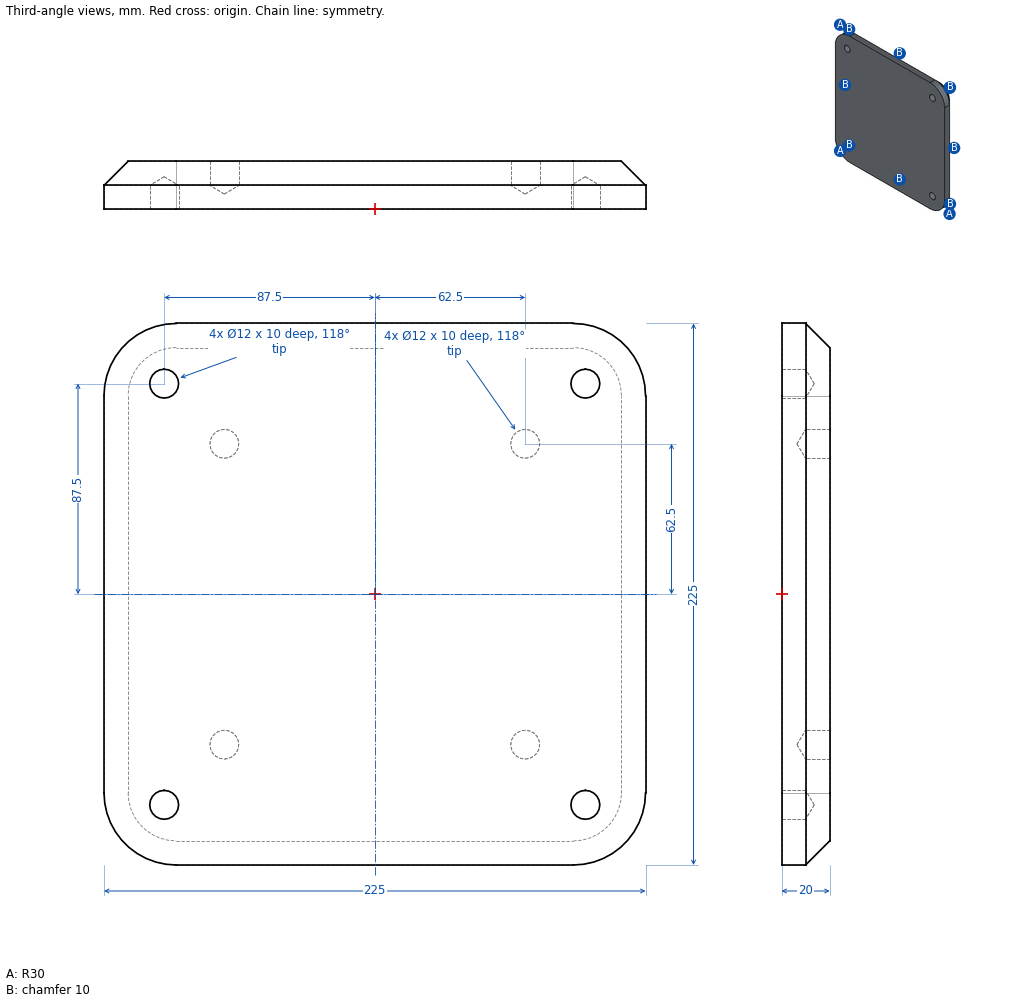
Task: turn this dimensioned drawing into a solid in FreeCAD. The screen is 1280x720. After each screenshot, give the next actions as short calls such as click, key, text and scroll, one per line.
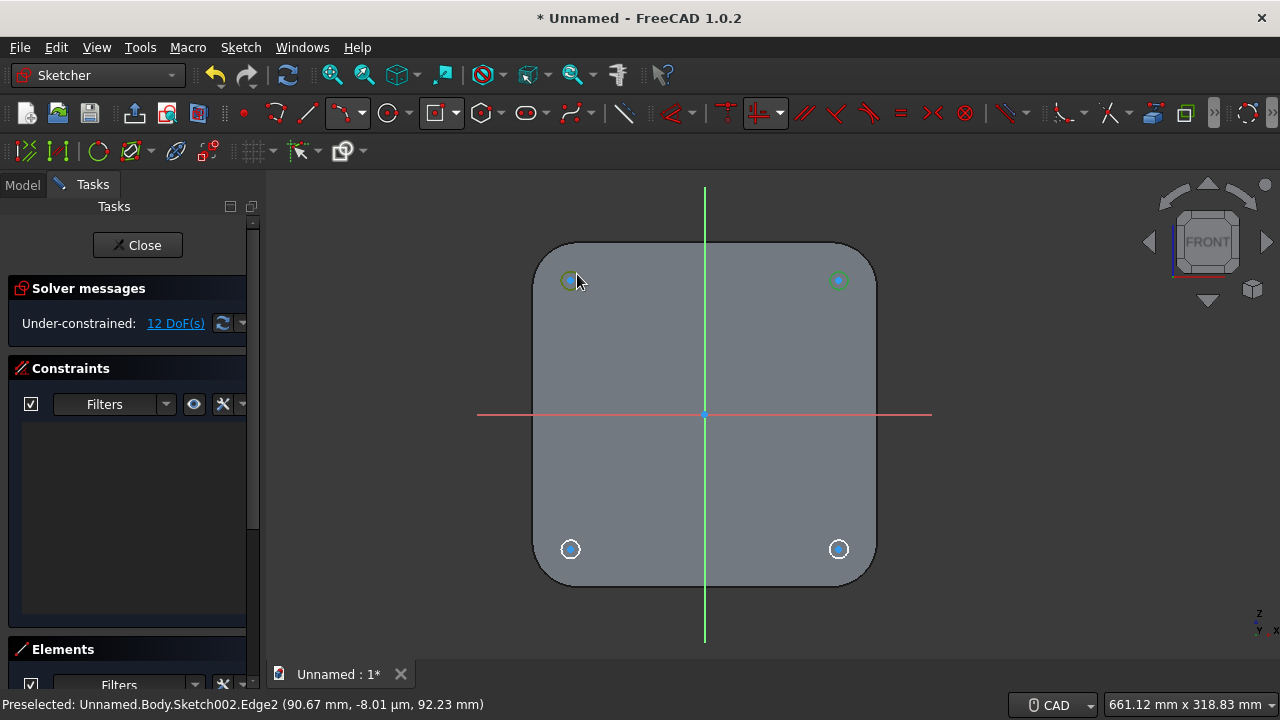
scroll(845, 543, up, 3)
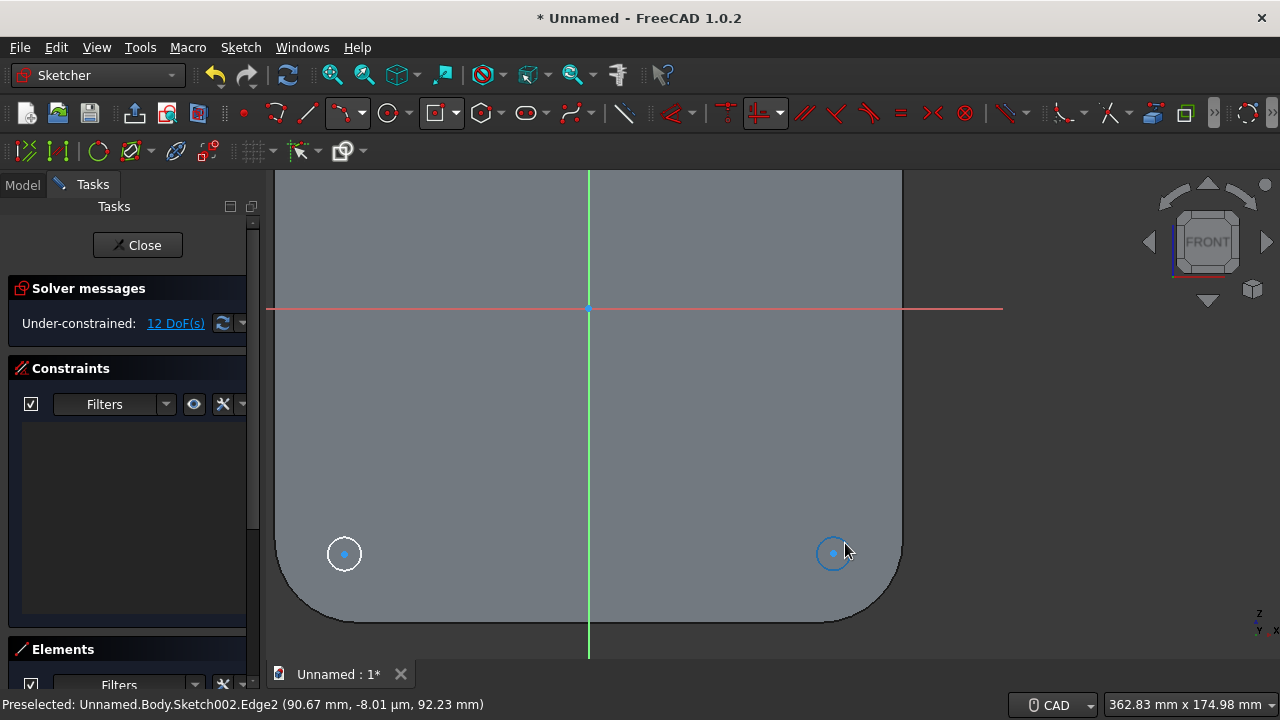
click(845, 542)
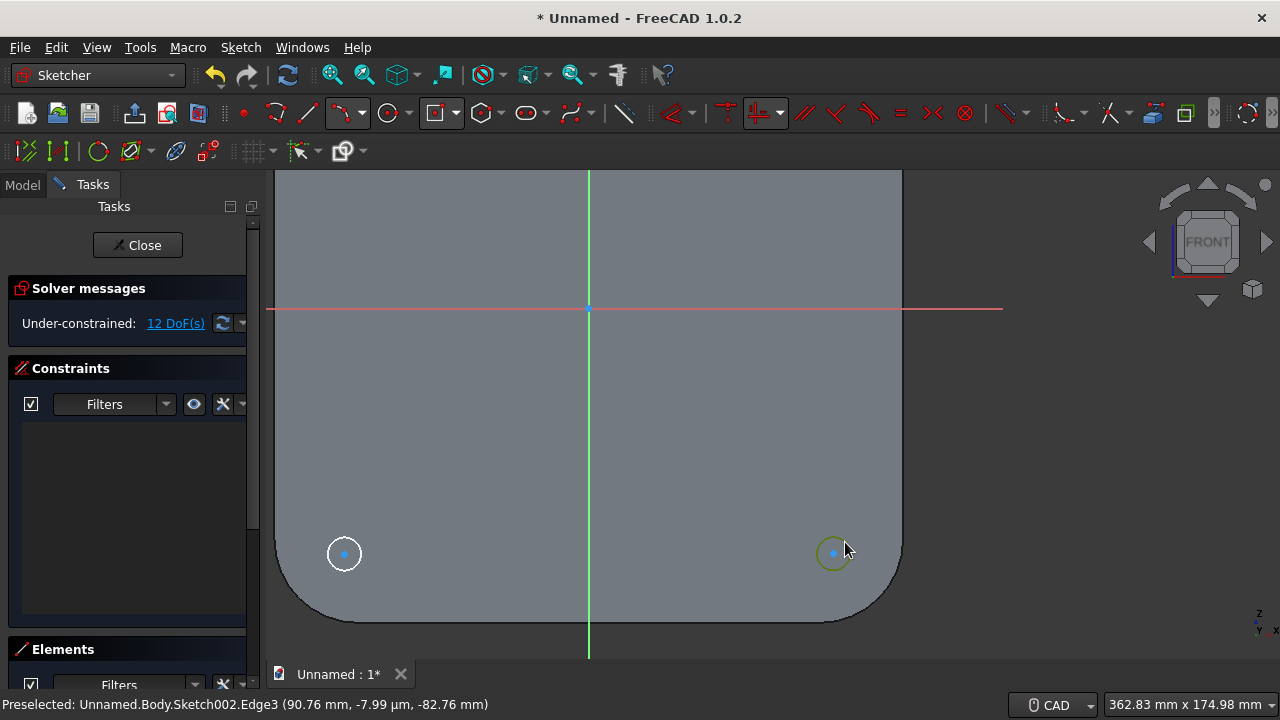
click(356, 542)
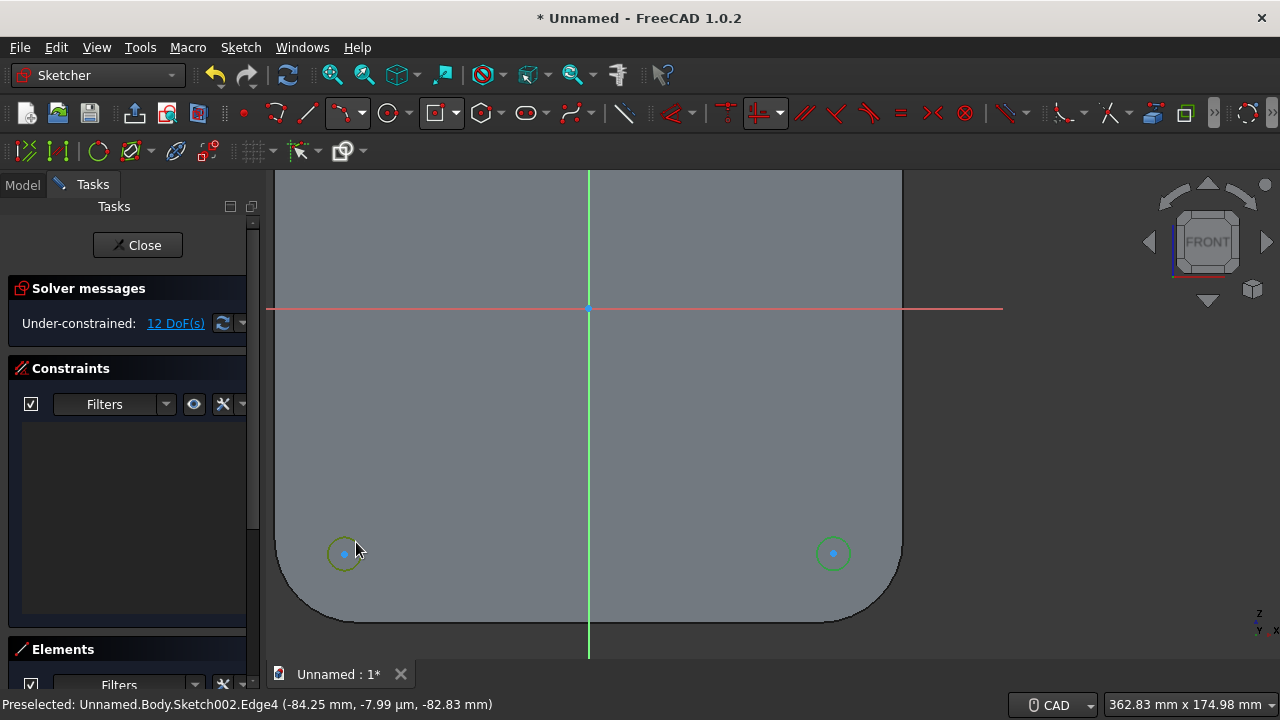
key(e)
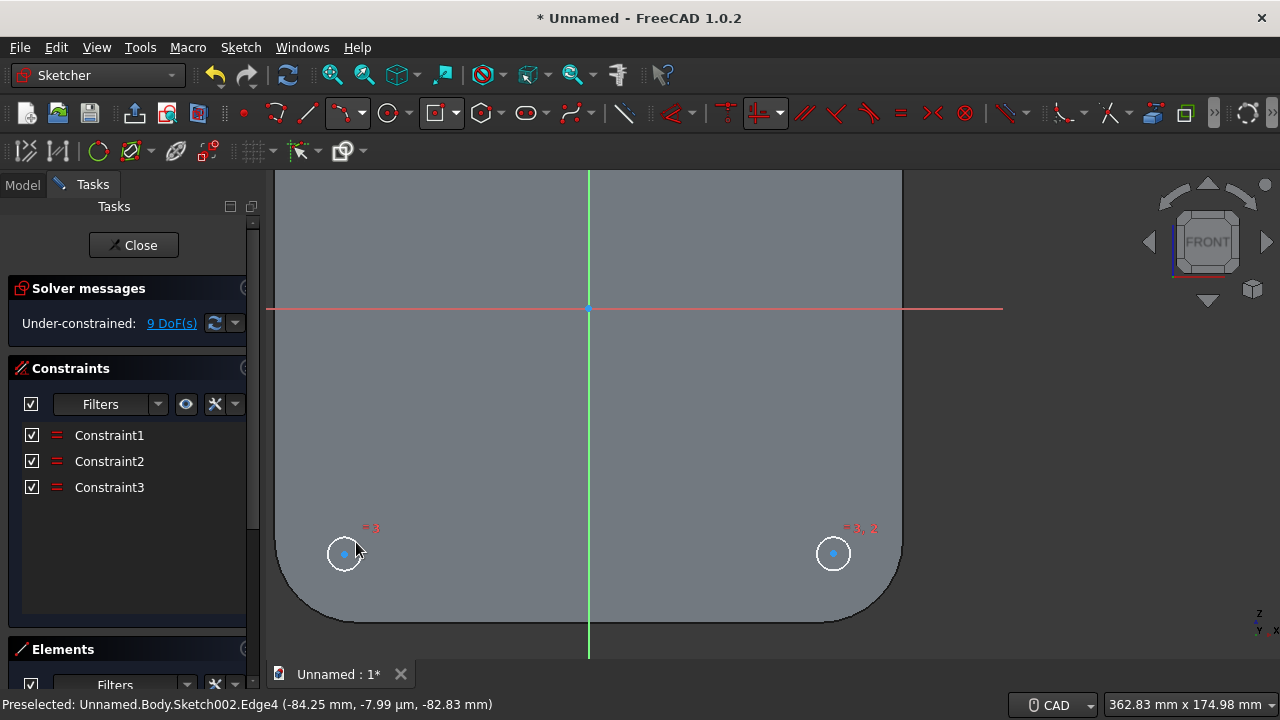
scroll(845, 543, down, 3)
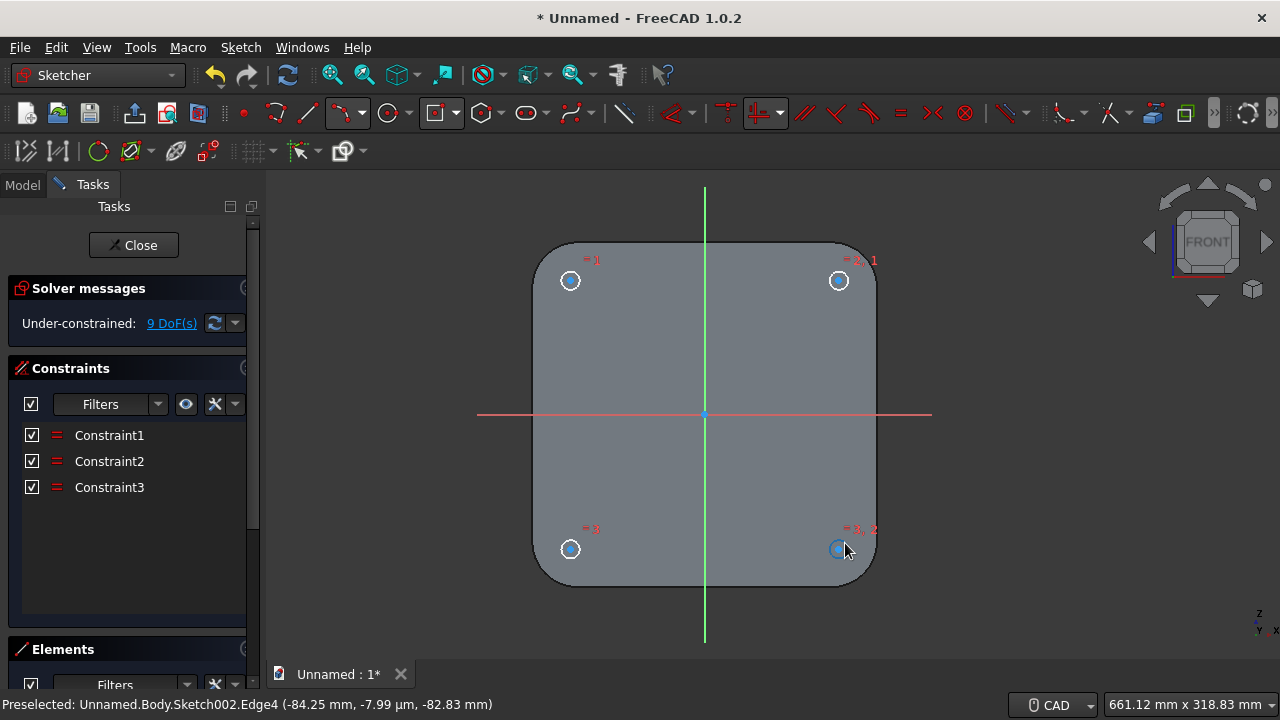
click(571, 281)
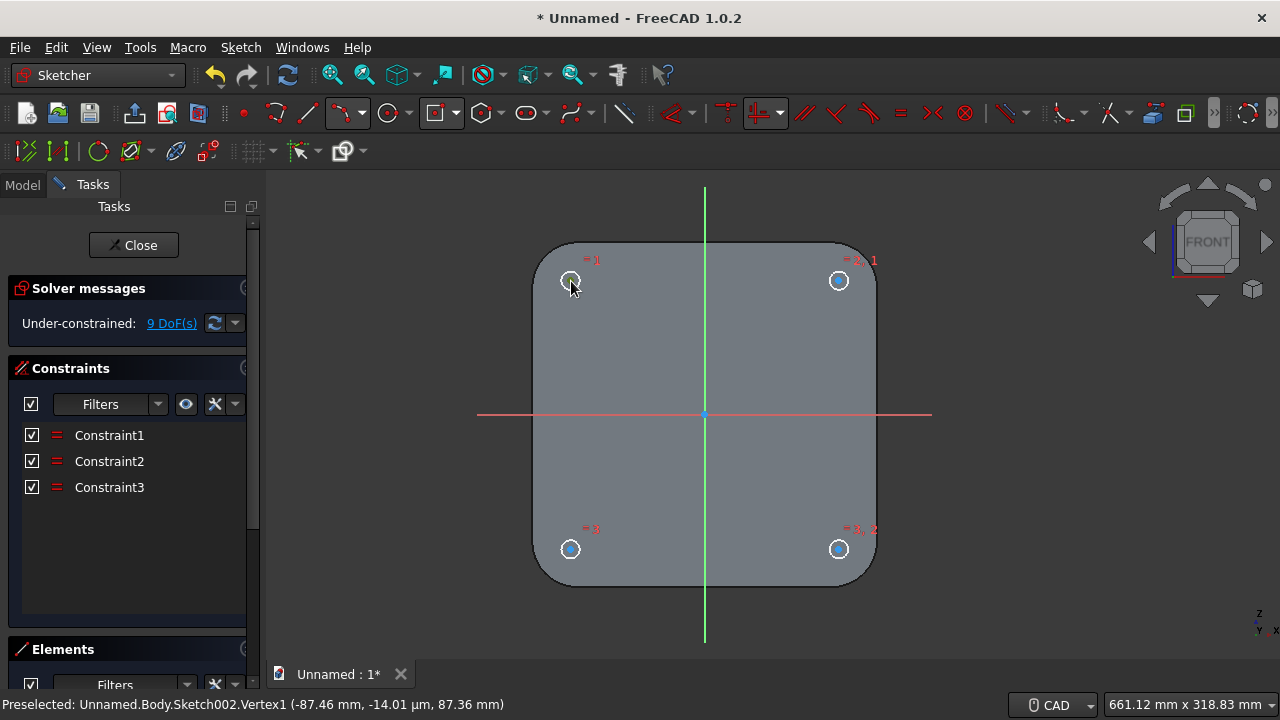
click(839, 281)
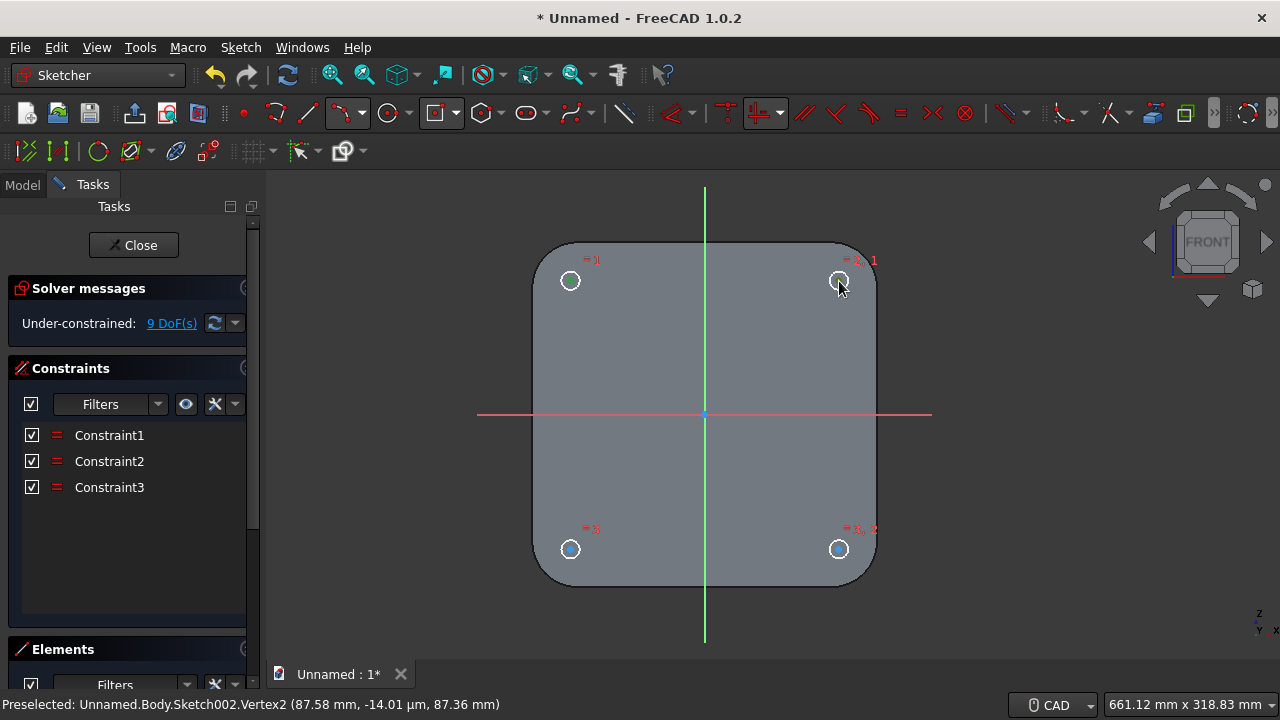
click(705, 600)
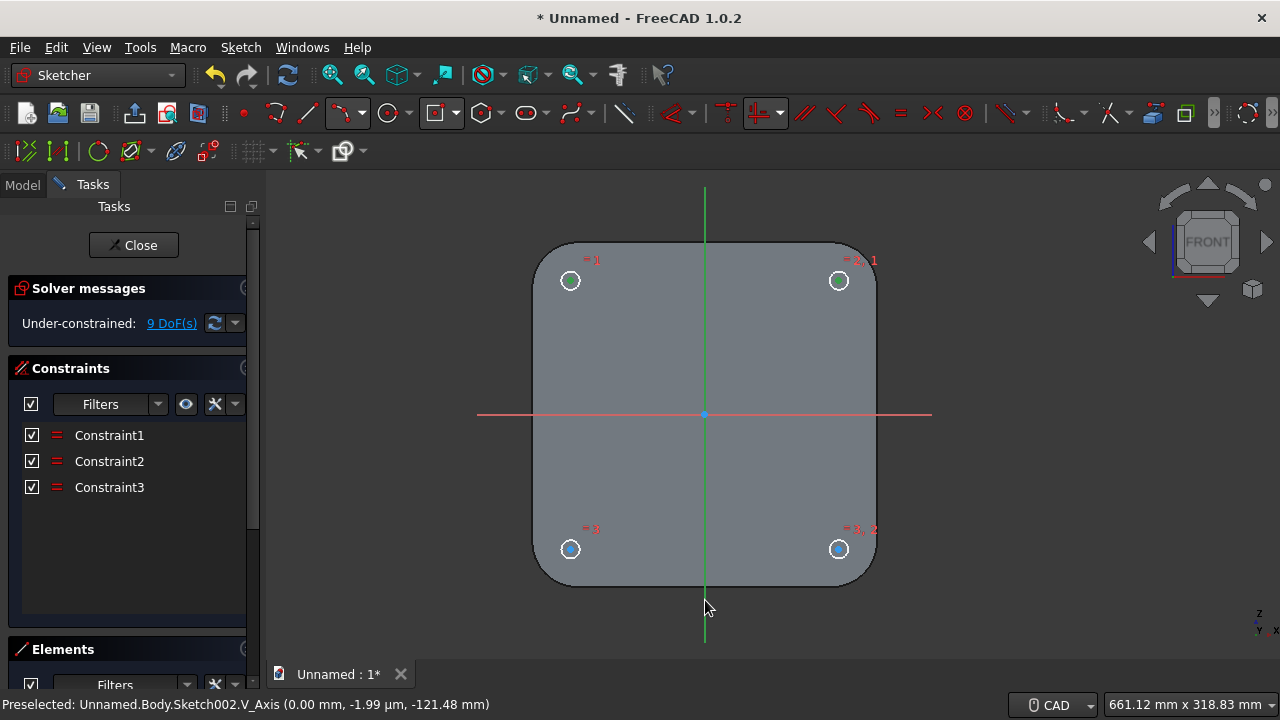
click(934, 114)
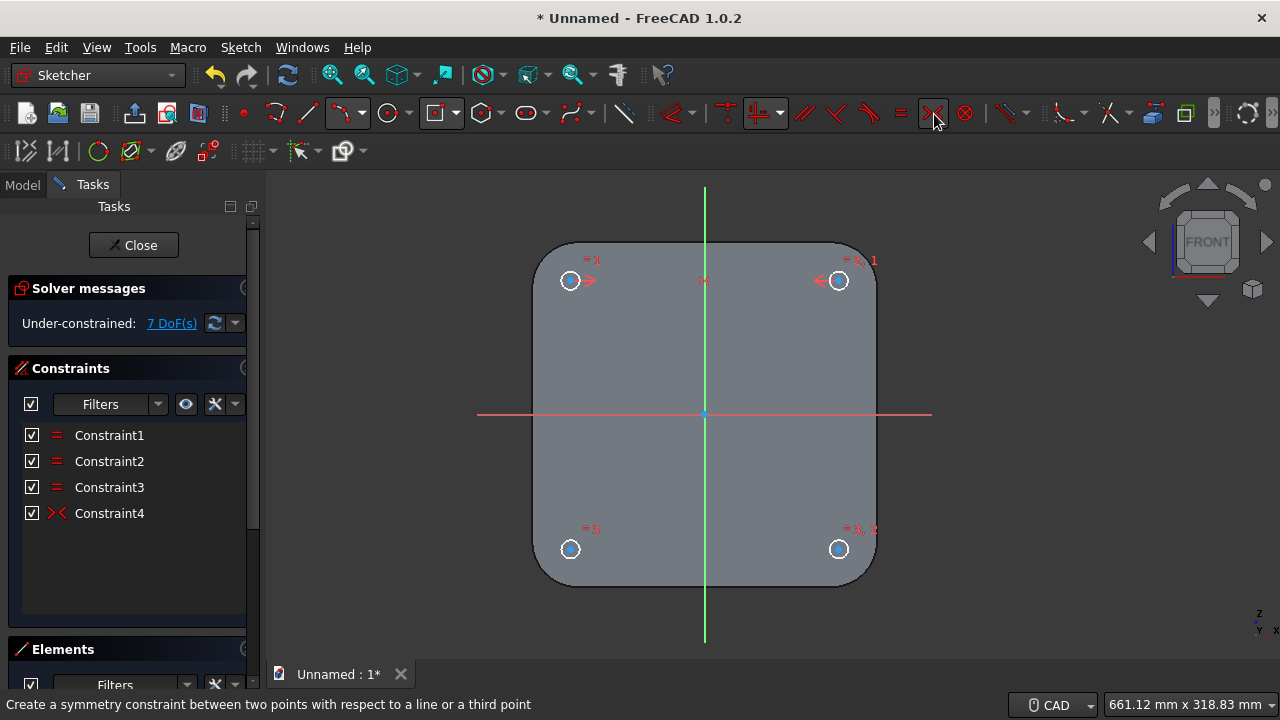
click(839, 281)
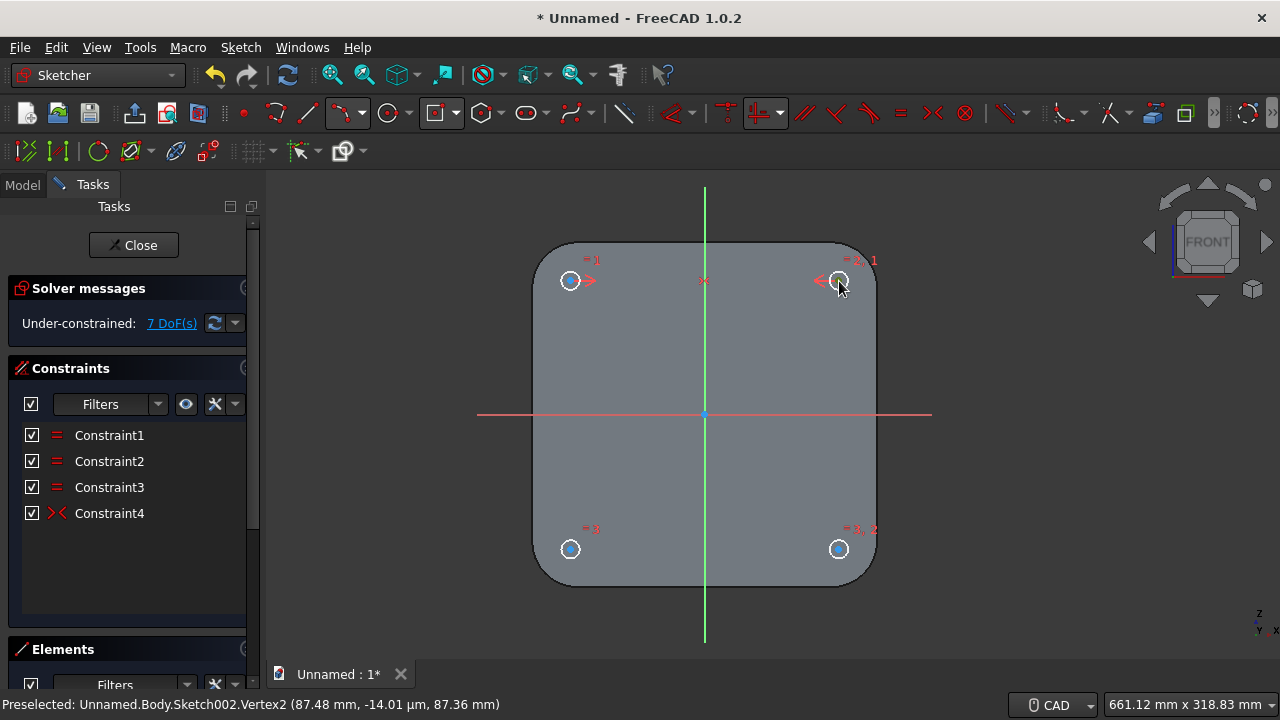
click(839, 549)